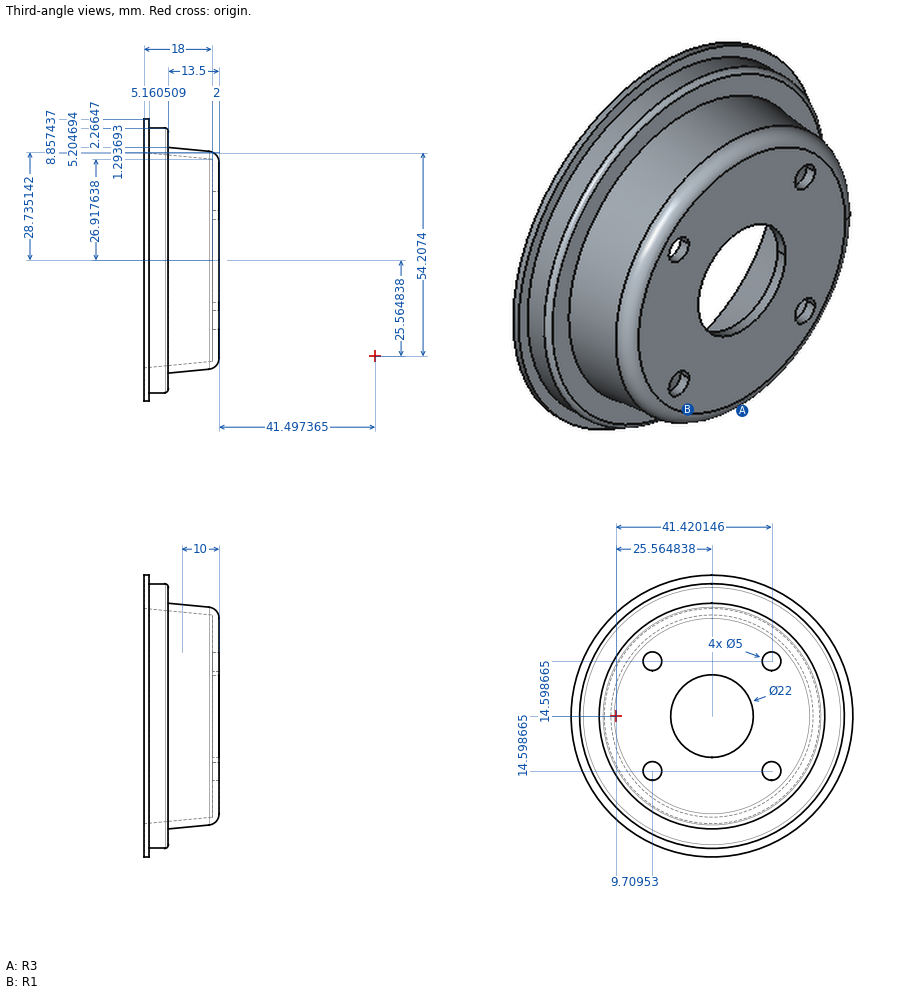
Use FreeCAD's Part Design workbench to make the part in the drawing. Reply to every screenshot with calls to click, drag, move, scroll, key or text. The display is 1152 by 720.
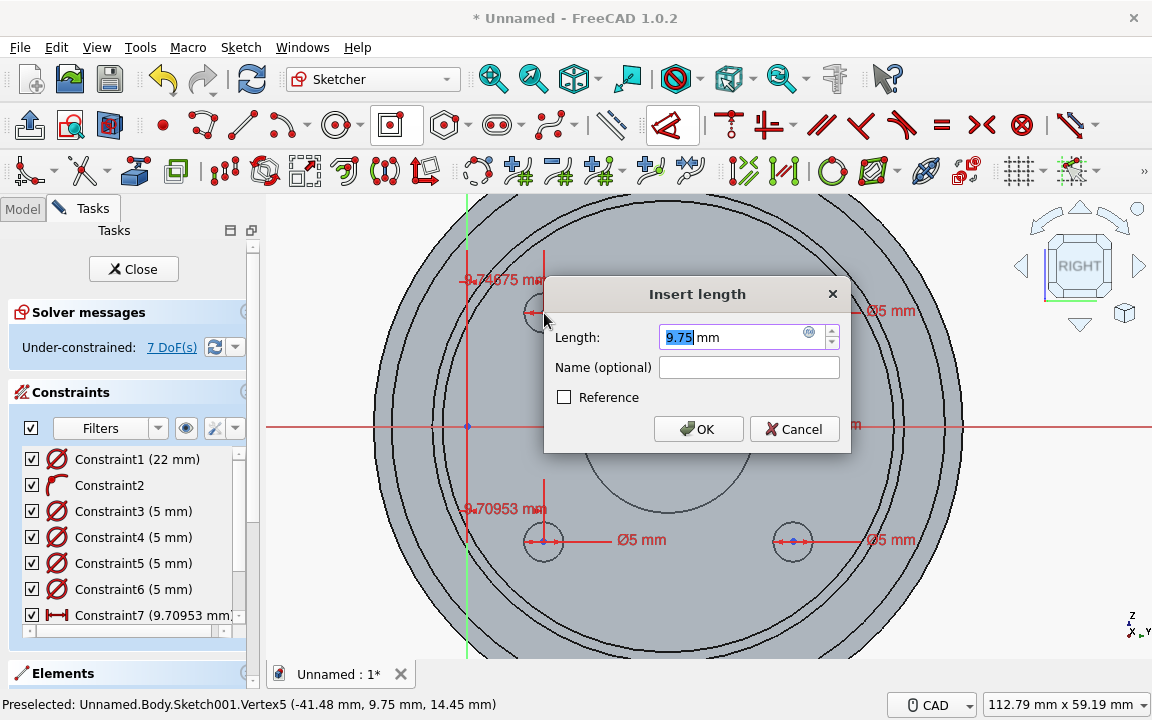
text(9.70953)
key(Return)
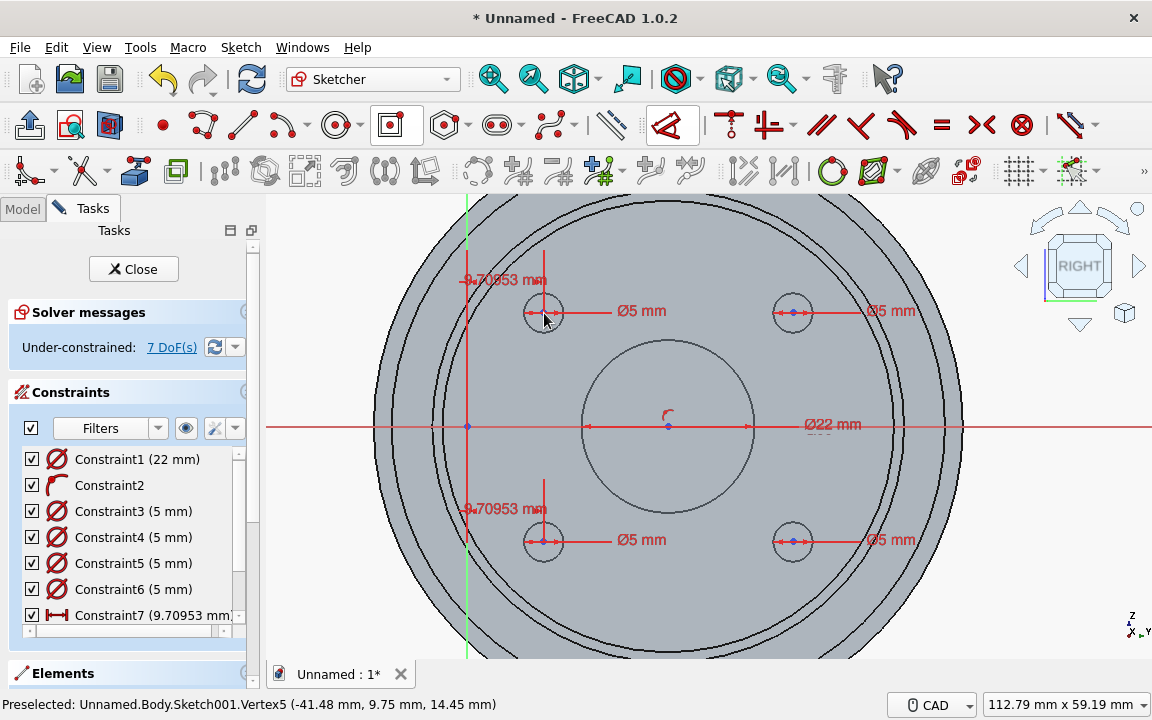
click(668, 426)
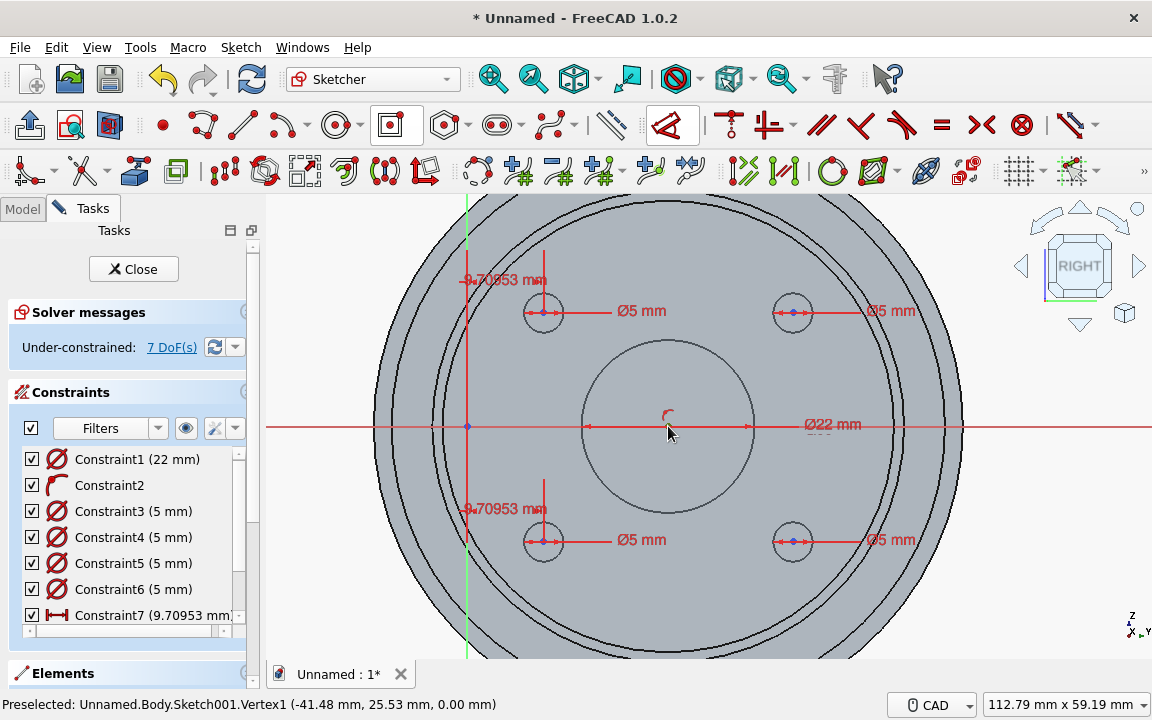
click(694, 126)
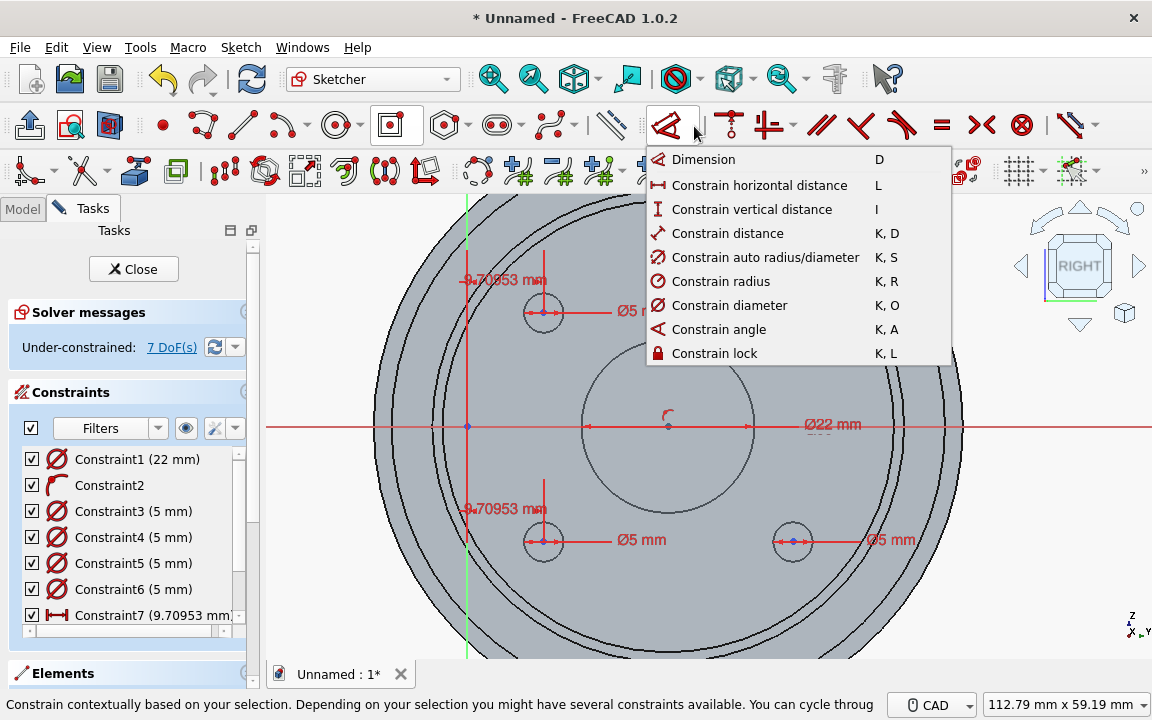
click(799, 185)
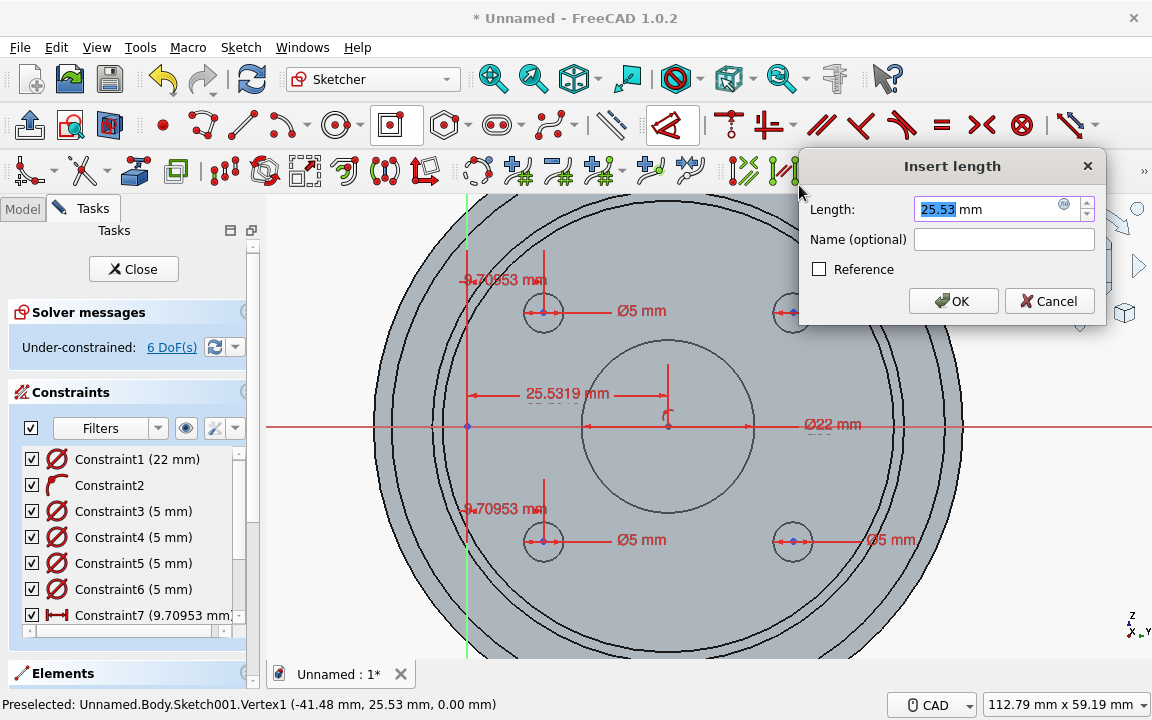
text(25.564838)
key(Return)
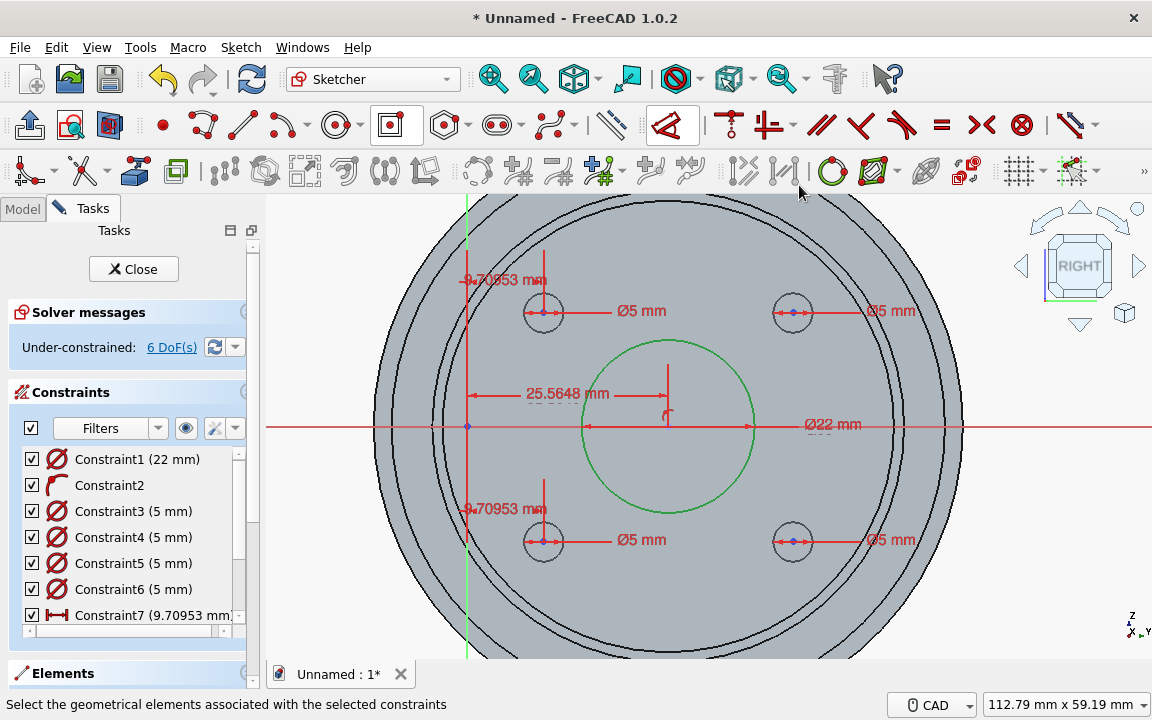
click(793, 313)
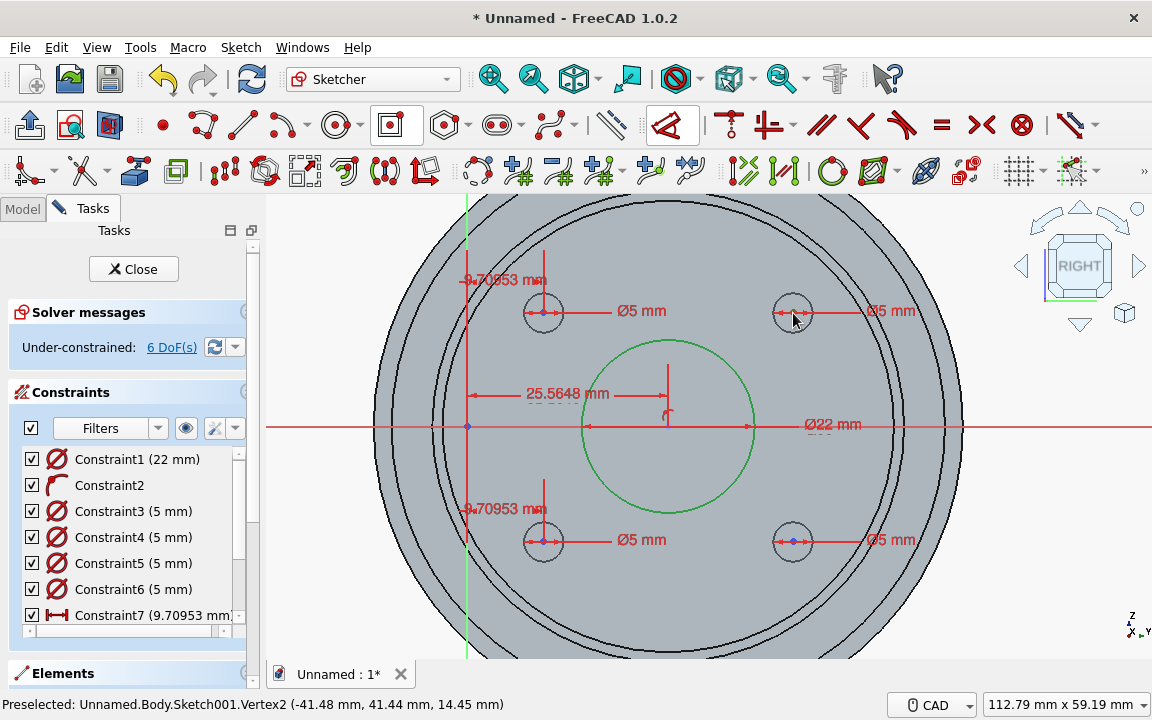
key(l)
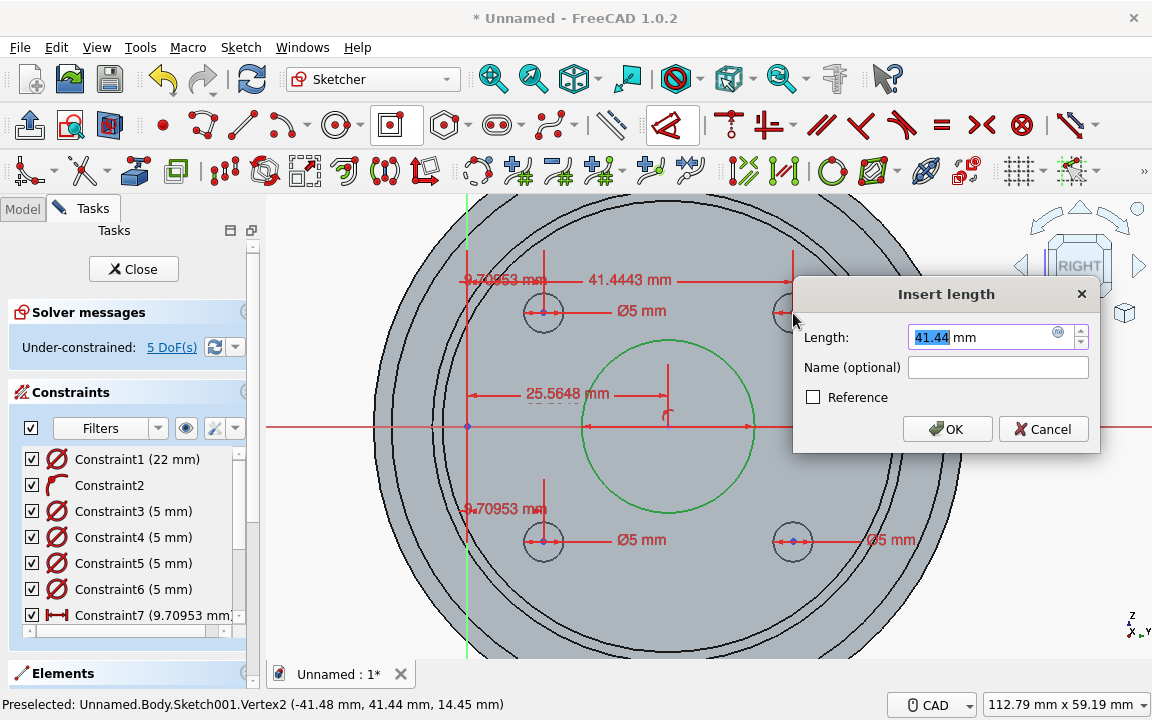
text(41.420146)
key(Return)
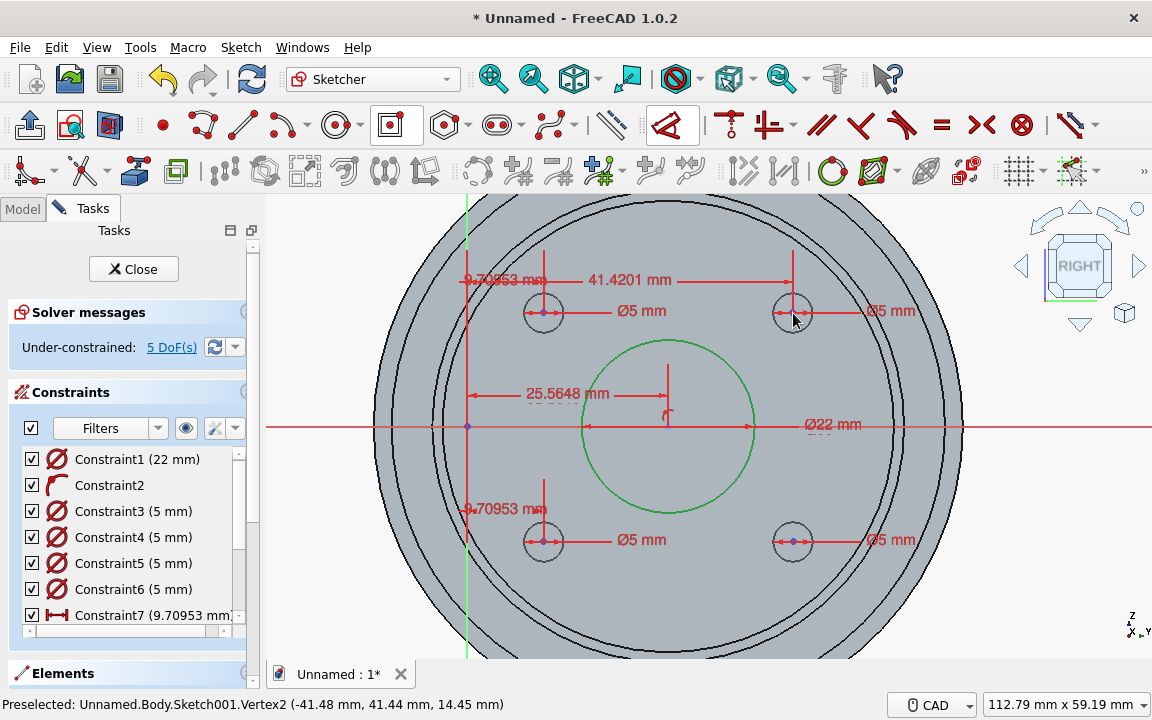
click(793, 313)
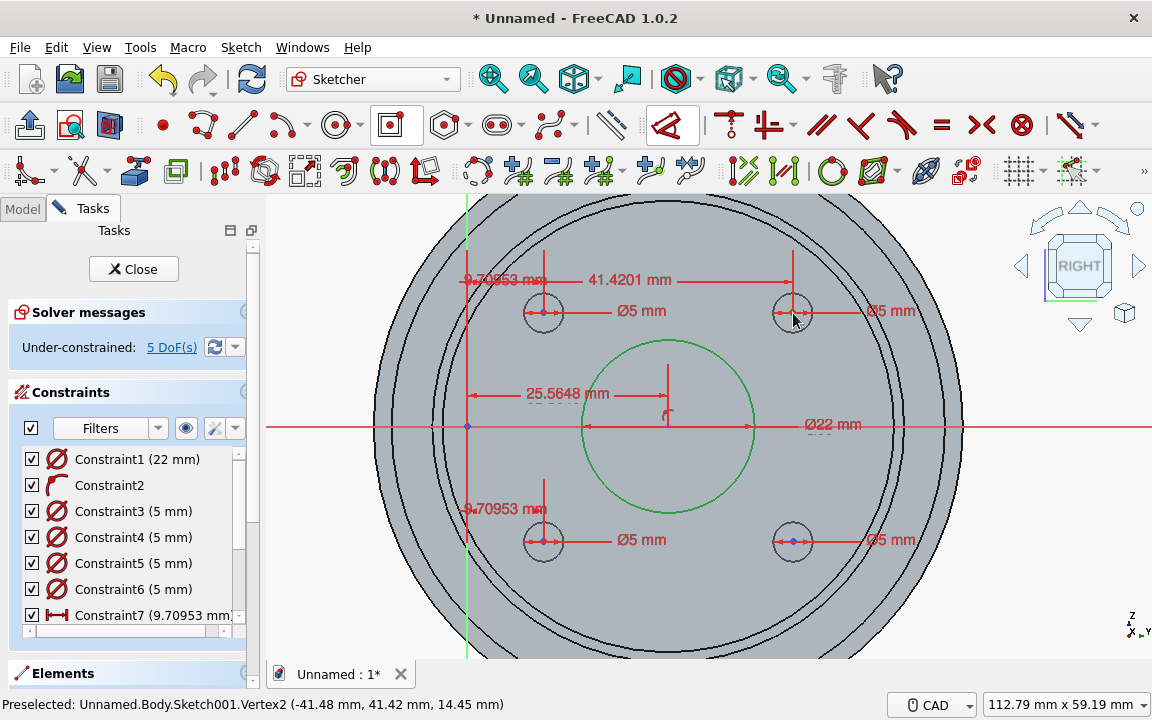
click(694, 126)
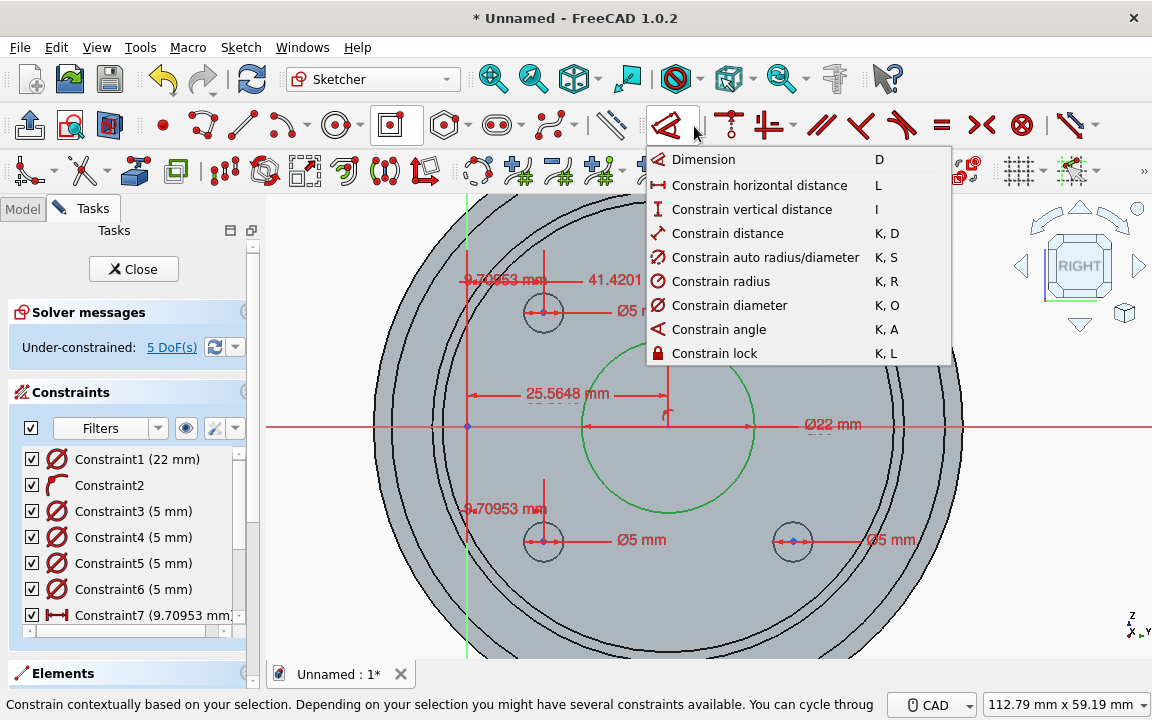
click(799, 209)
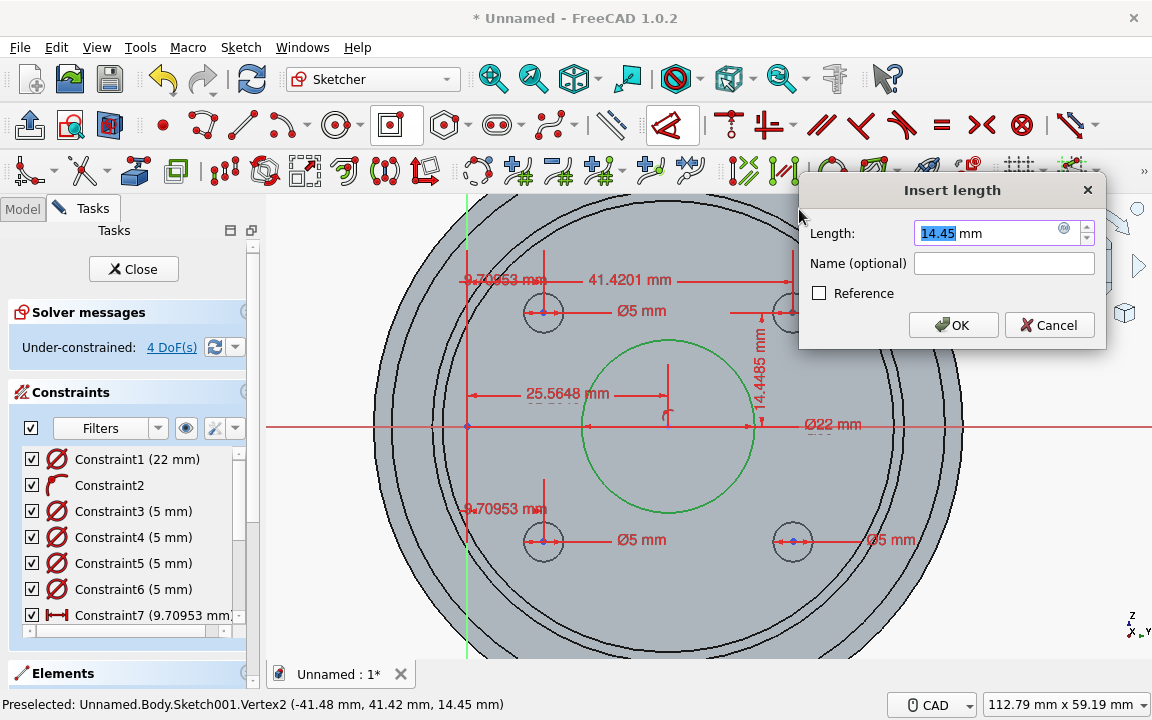
text(14.598665)
key(Return)